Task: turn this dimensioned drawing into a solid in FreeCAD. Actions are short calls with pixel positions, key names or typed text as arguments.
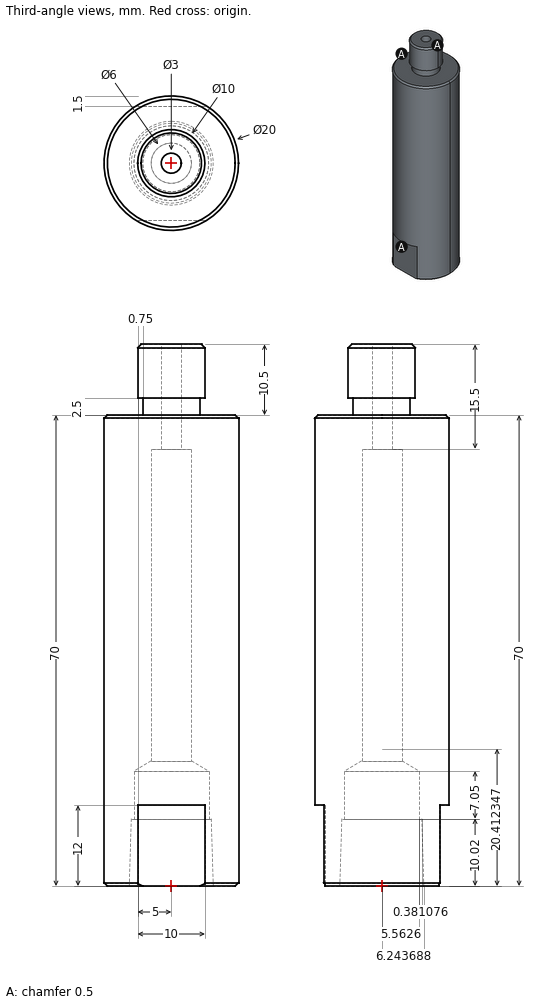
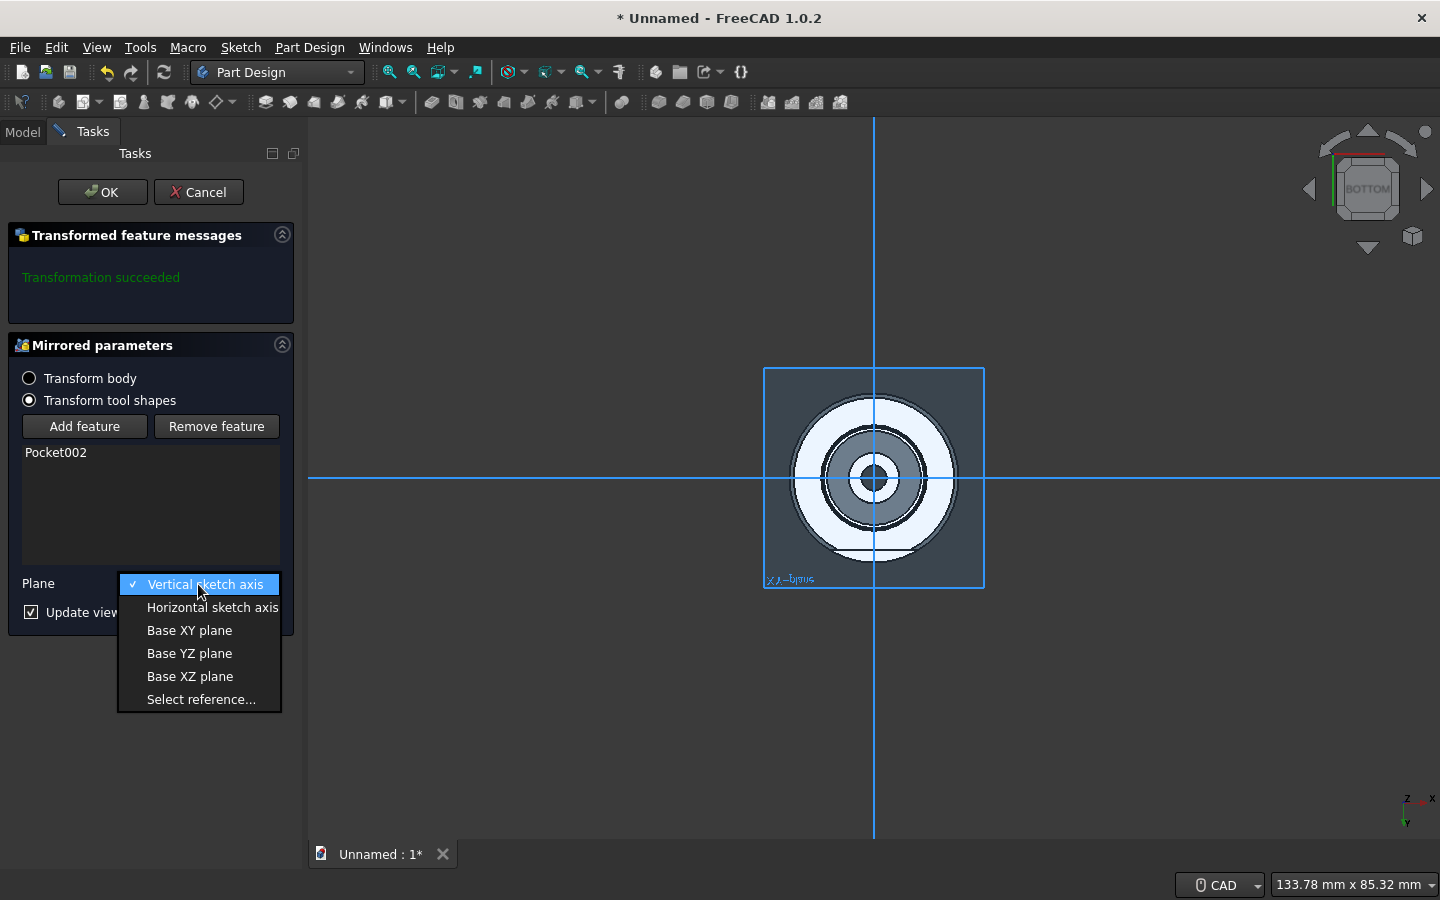
click(198, 676)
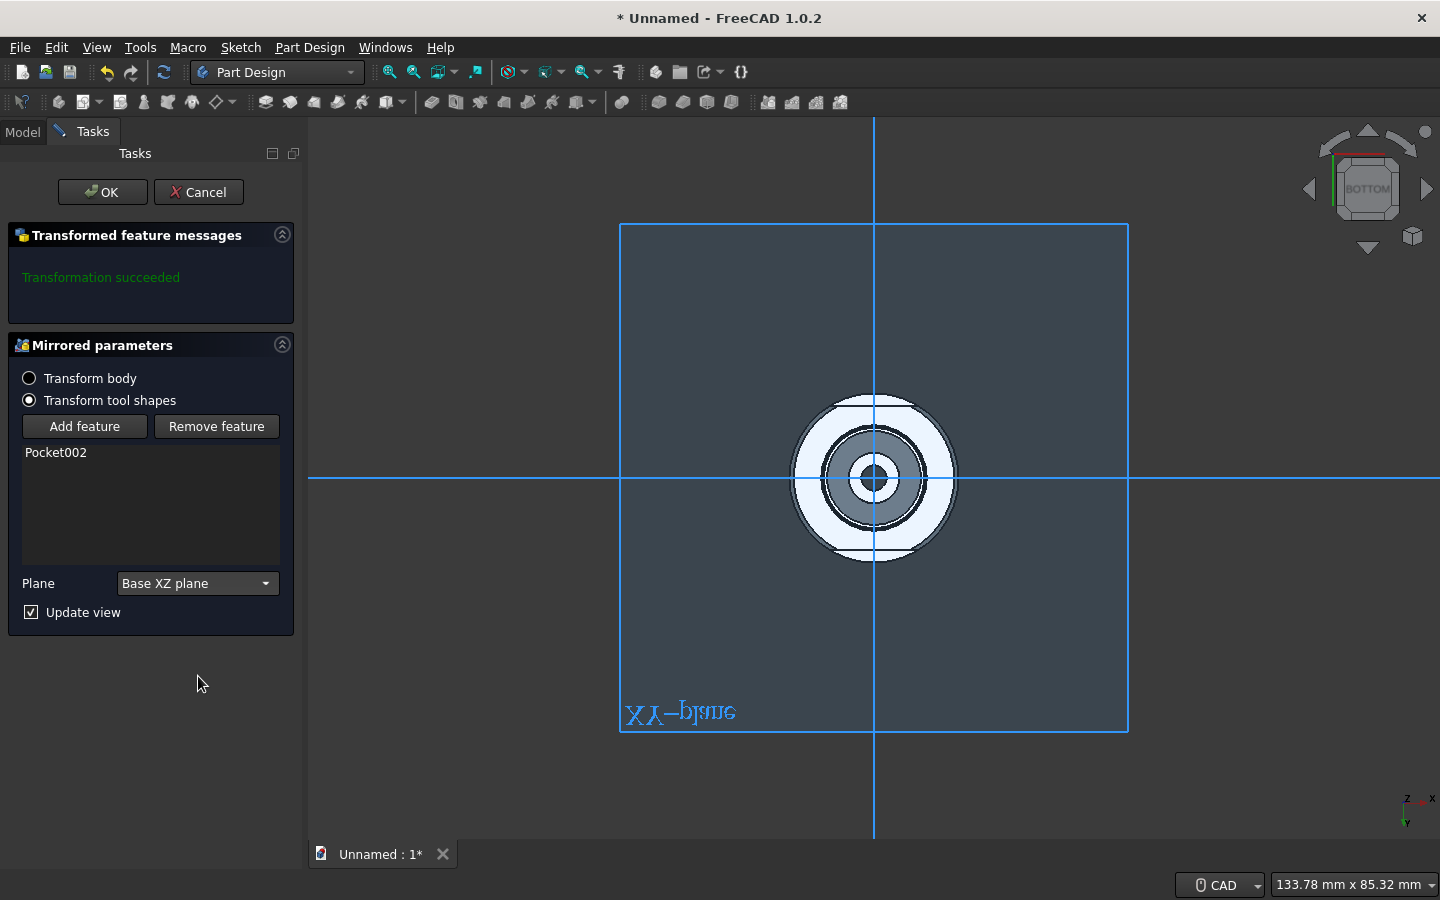
click(103, 192)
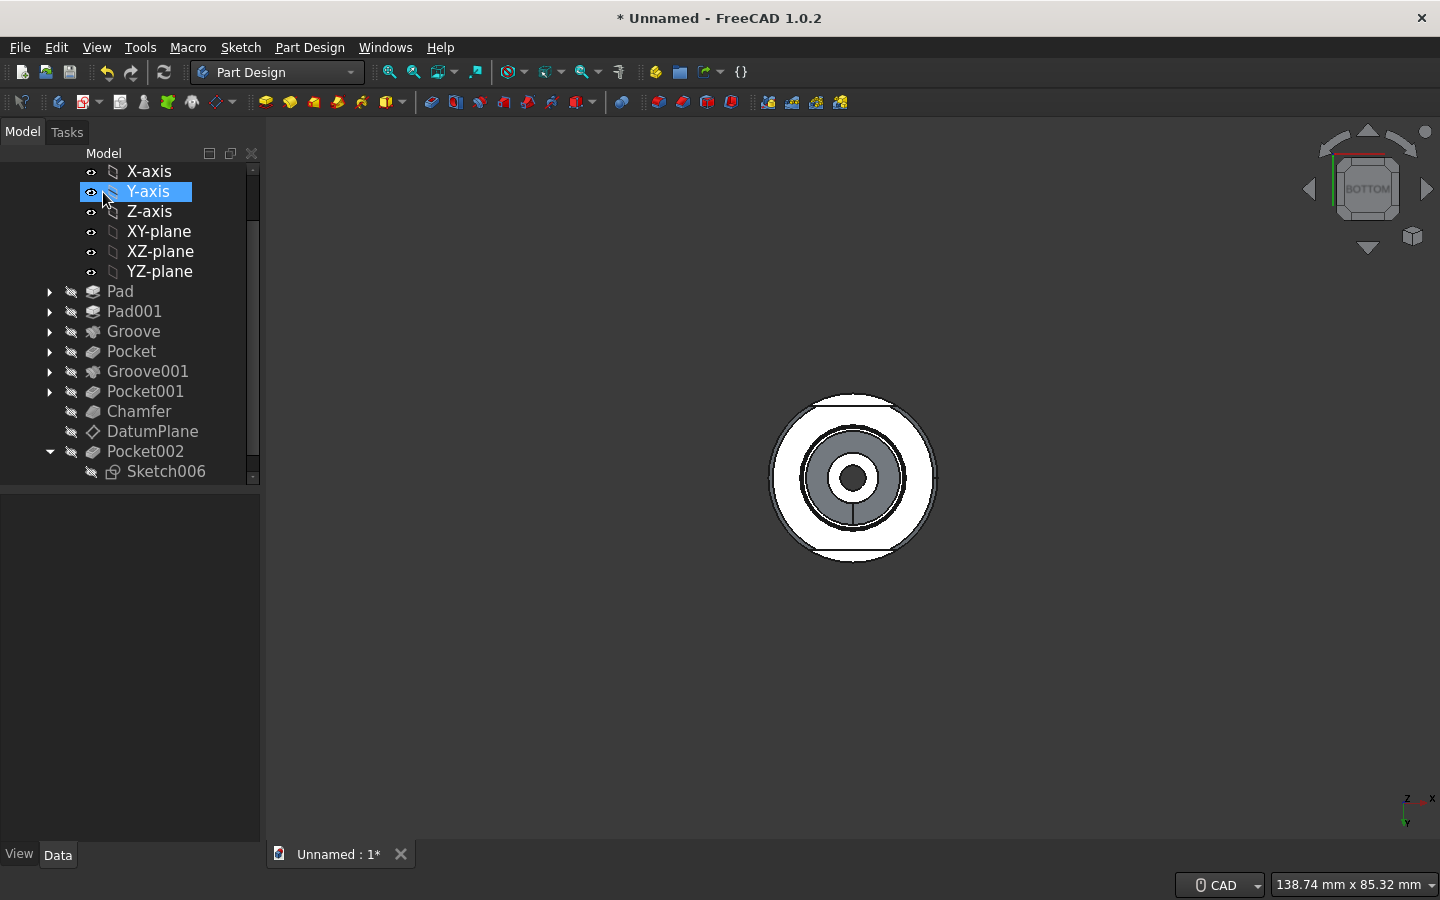
key(0)